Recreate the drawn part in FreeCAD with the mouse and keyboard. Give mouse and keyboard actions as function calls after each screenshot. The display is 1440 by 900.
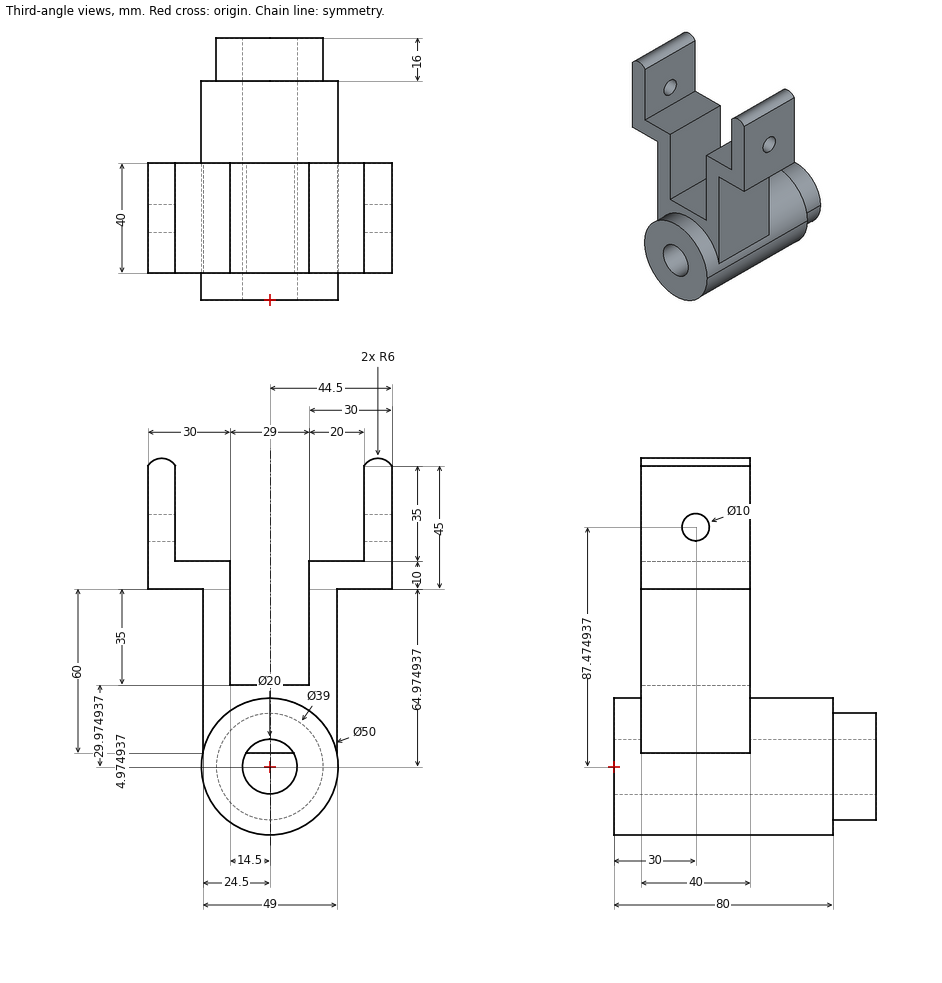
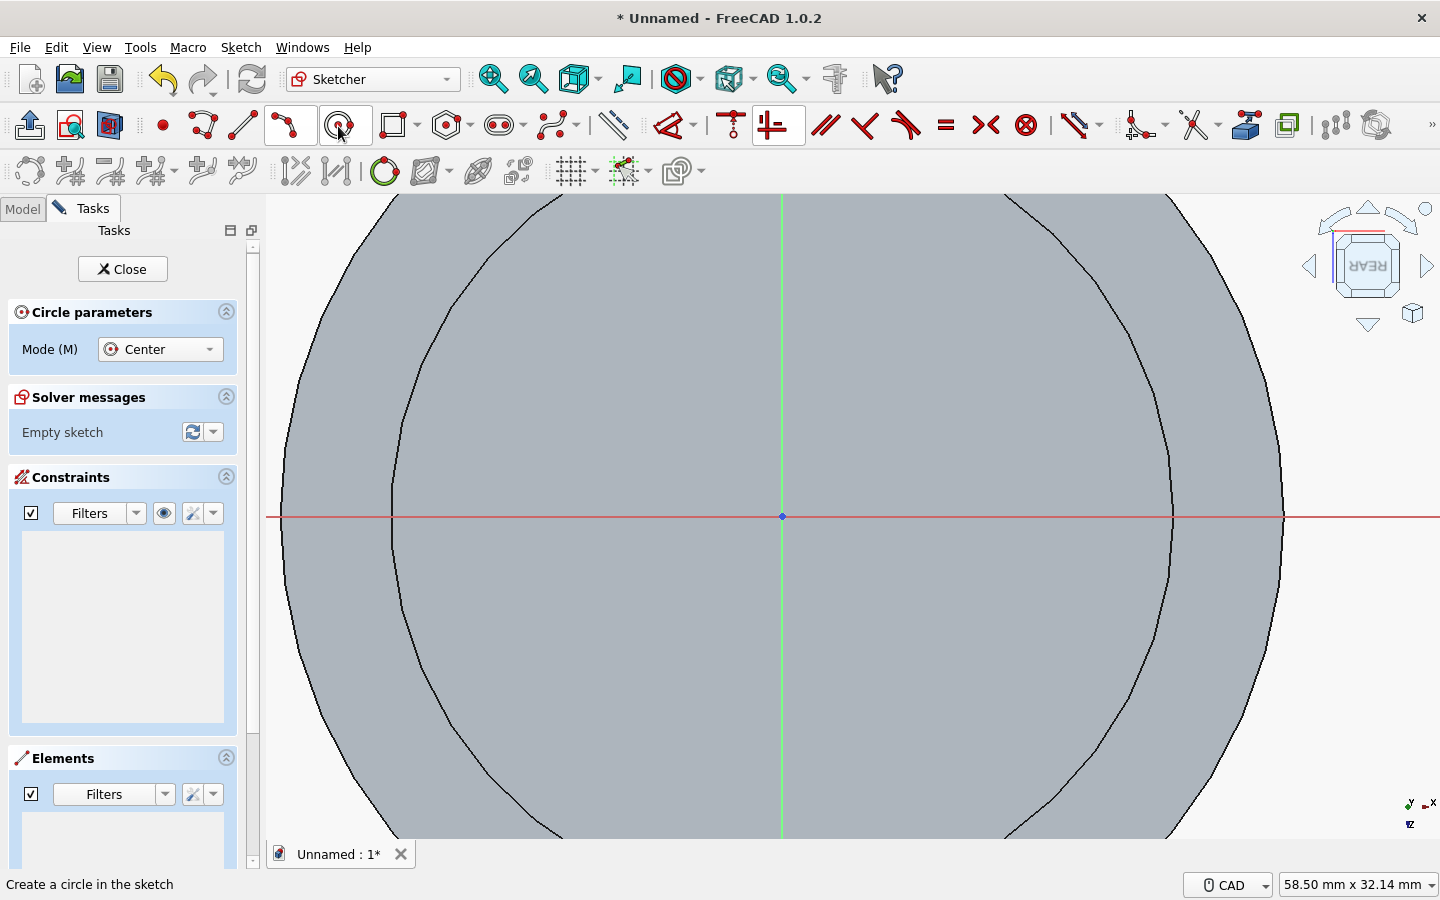
click(782, 516)
click(924, 375)
key(Escape)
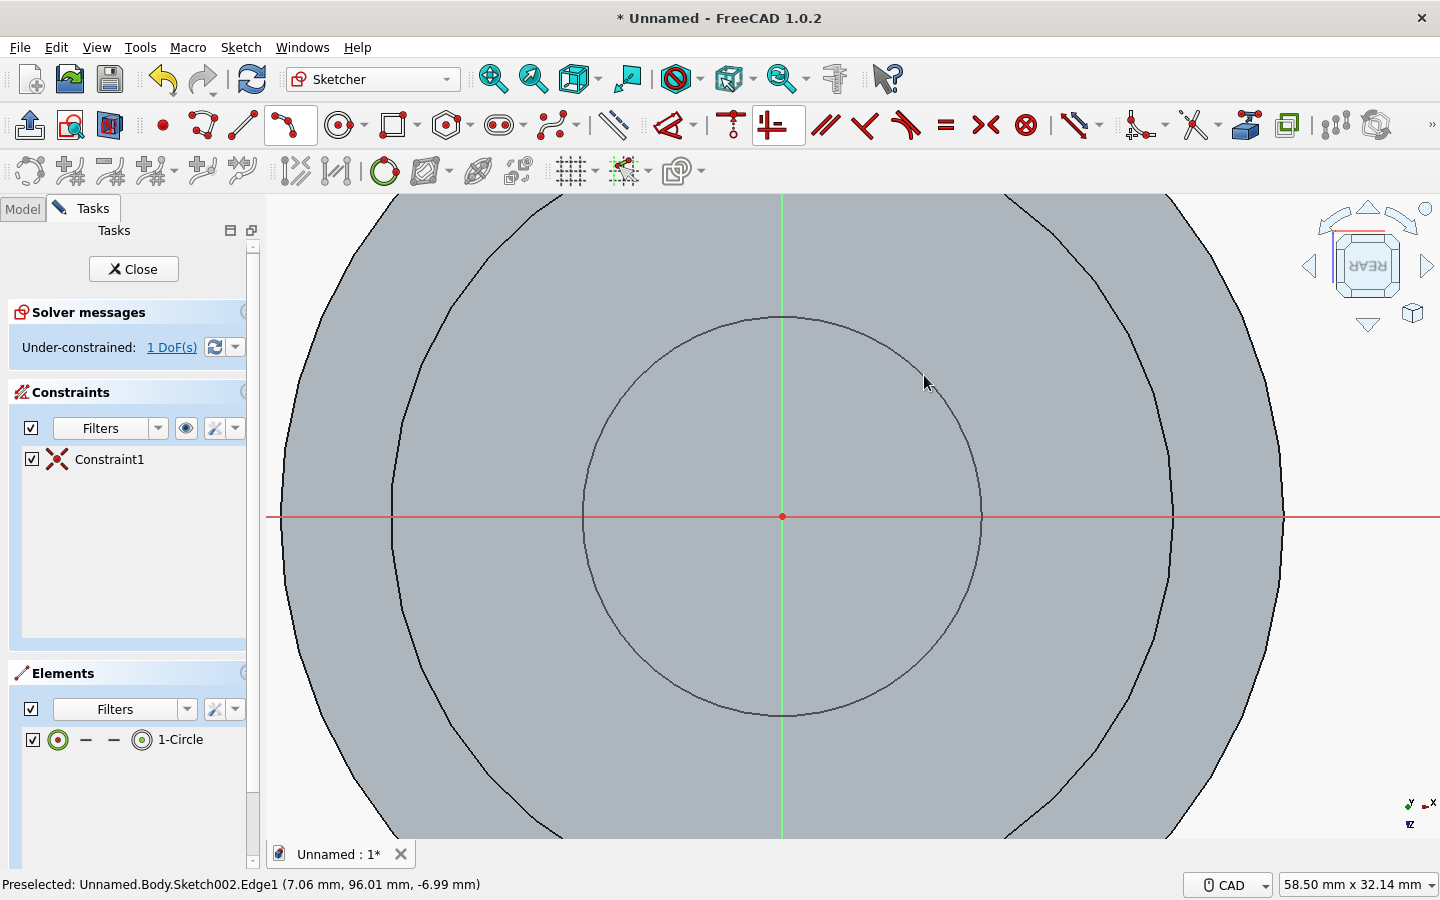
click(668, 126)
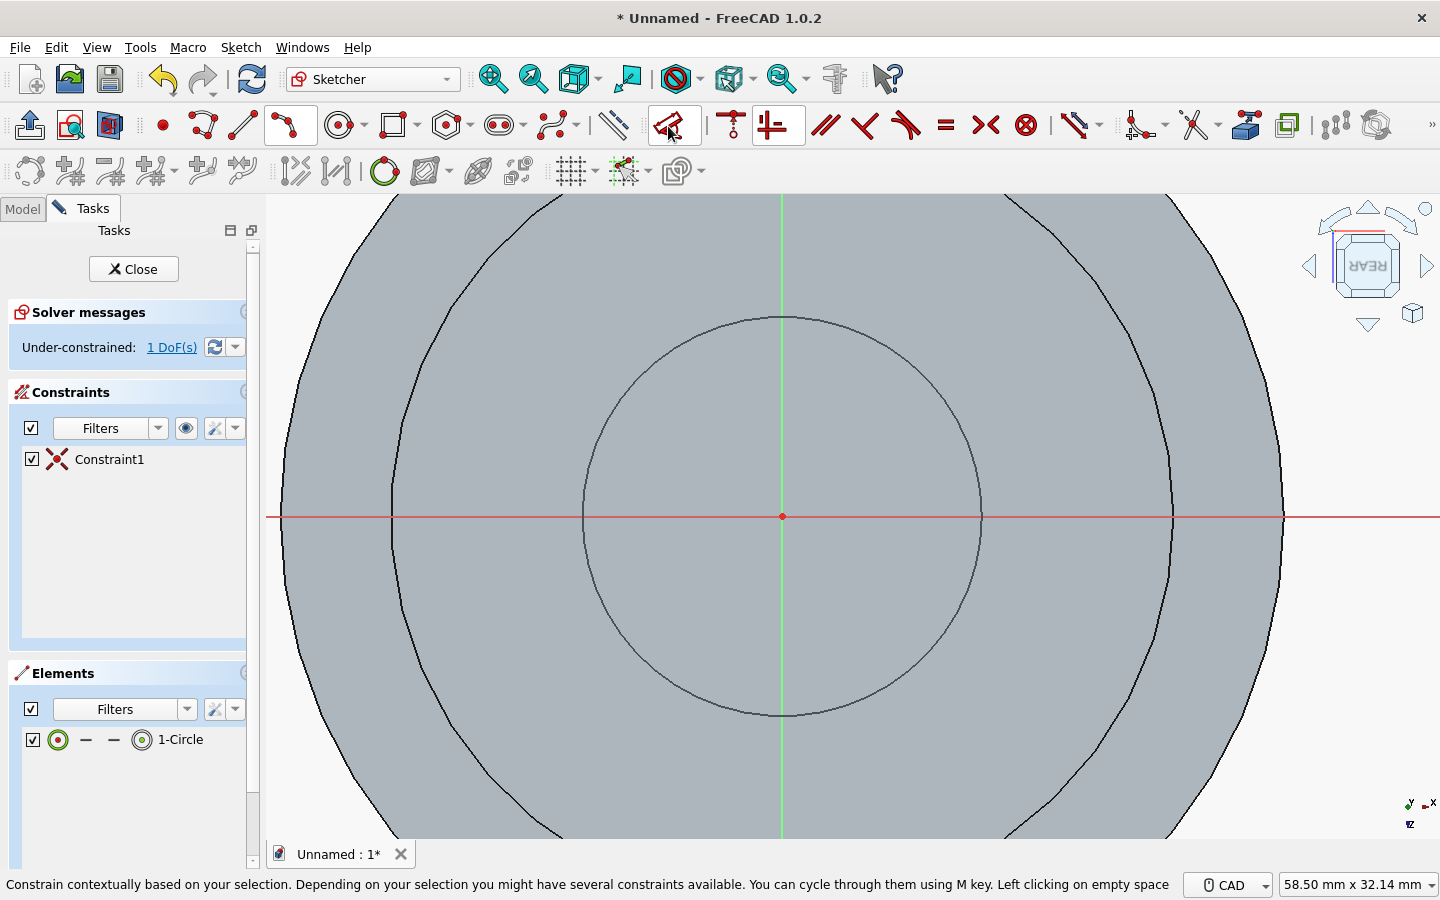
click(923, 375)
click(946, 352)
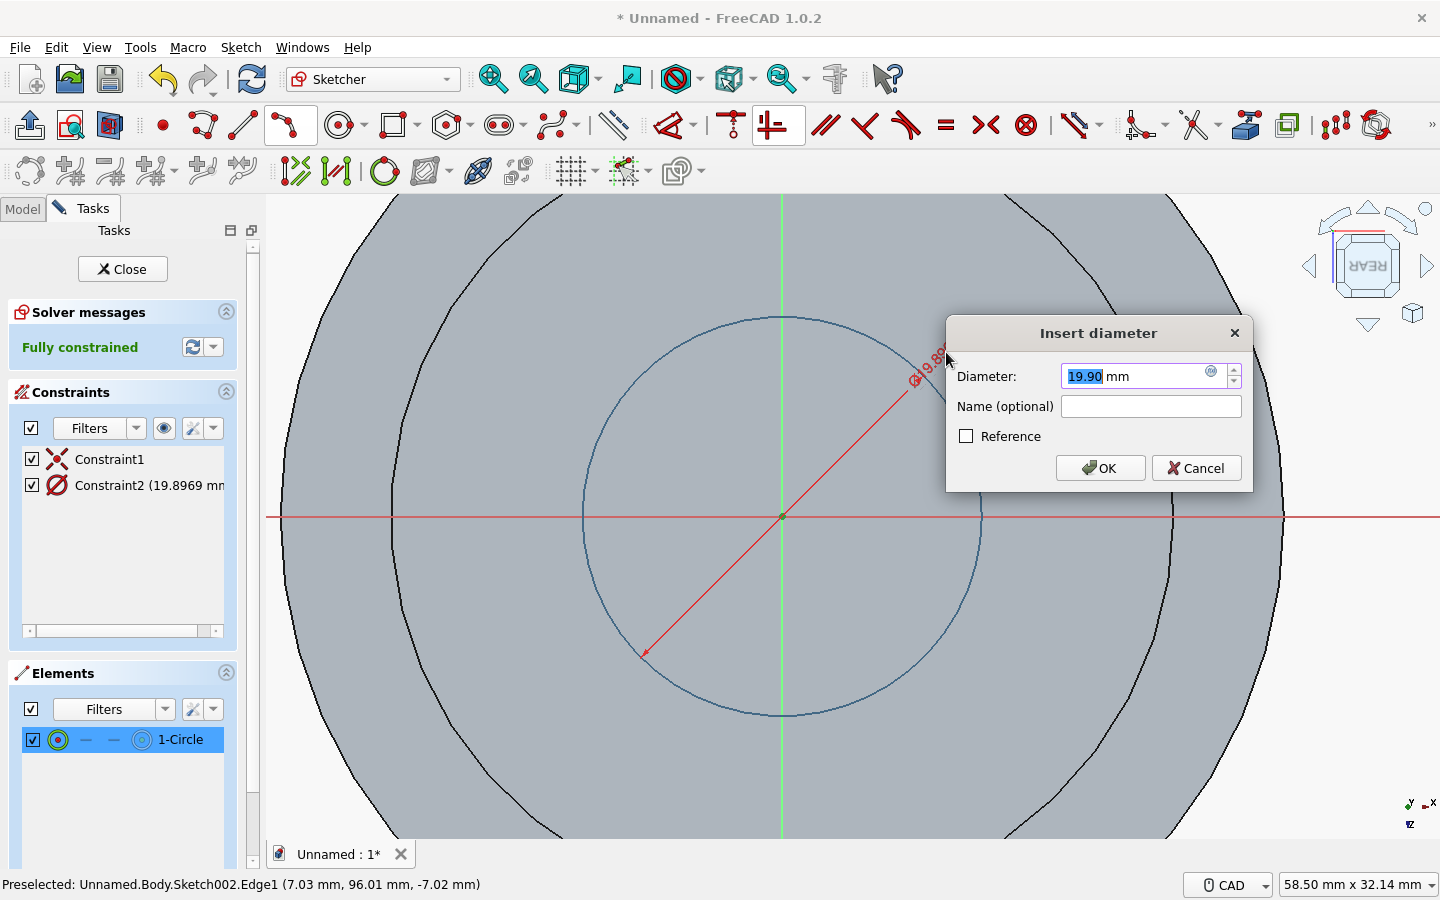
text(20)
key(Return)
key(Escape)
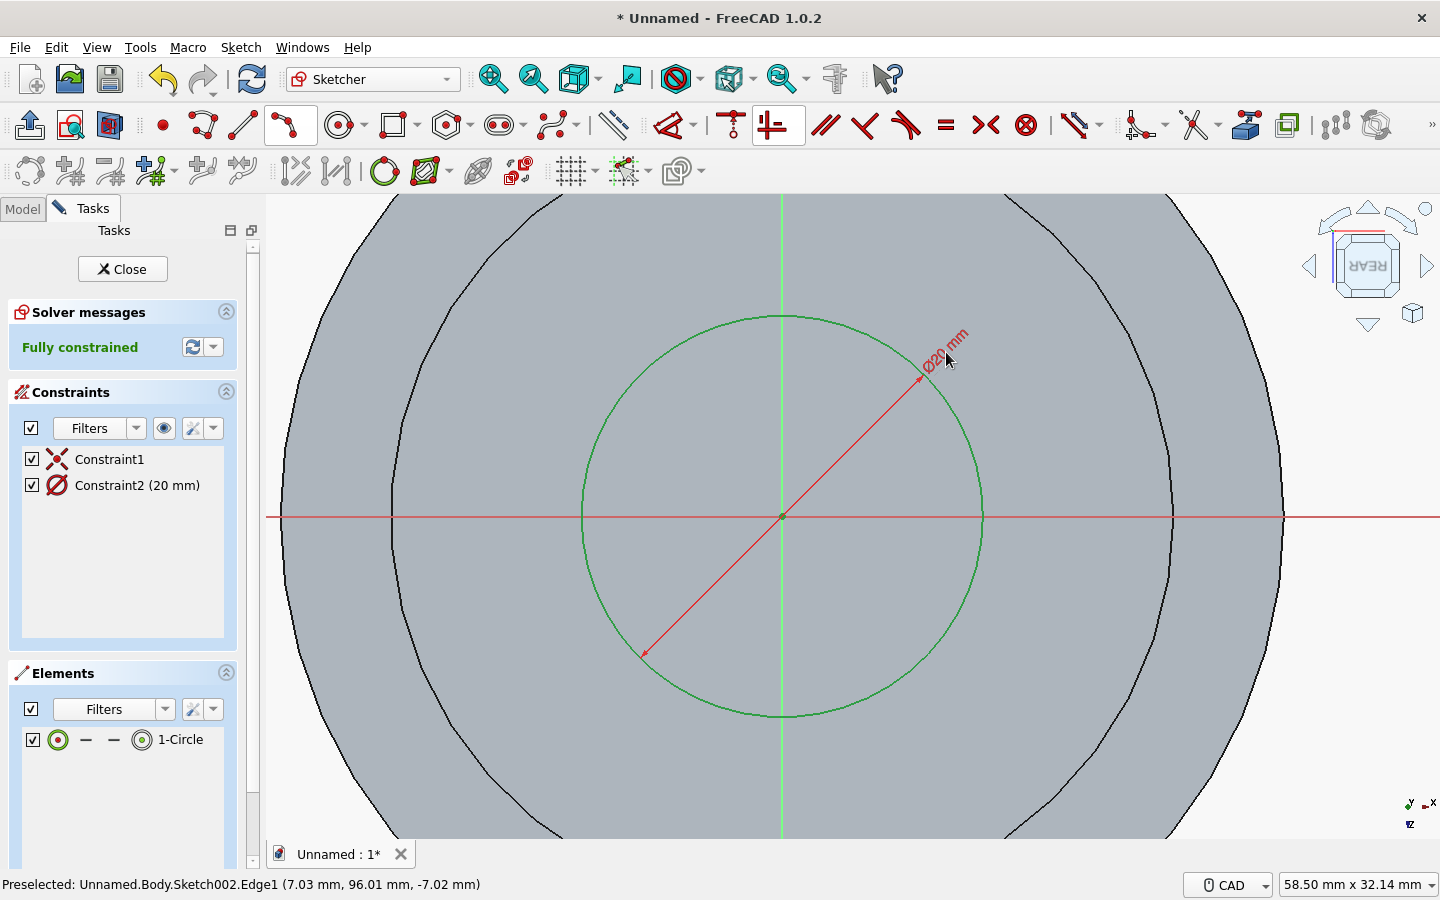
click(123, 269)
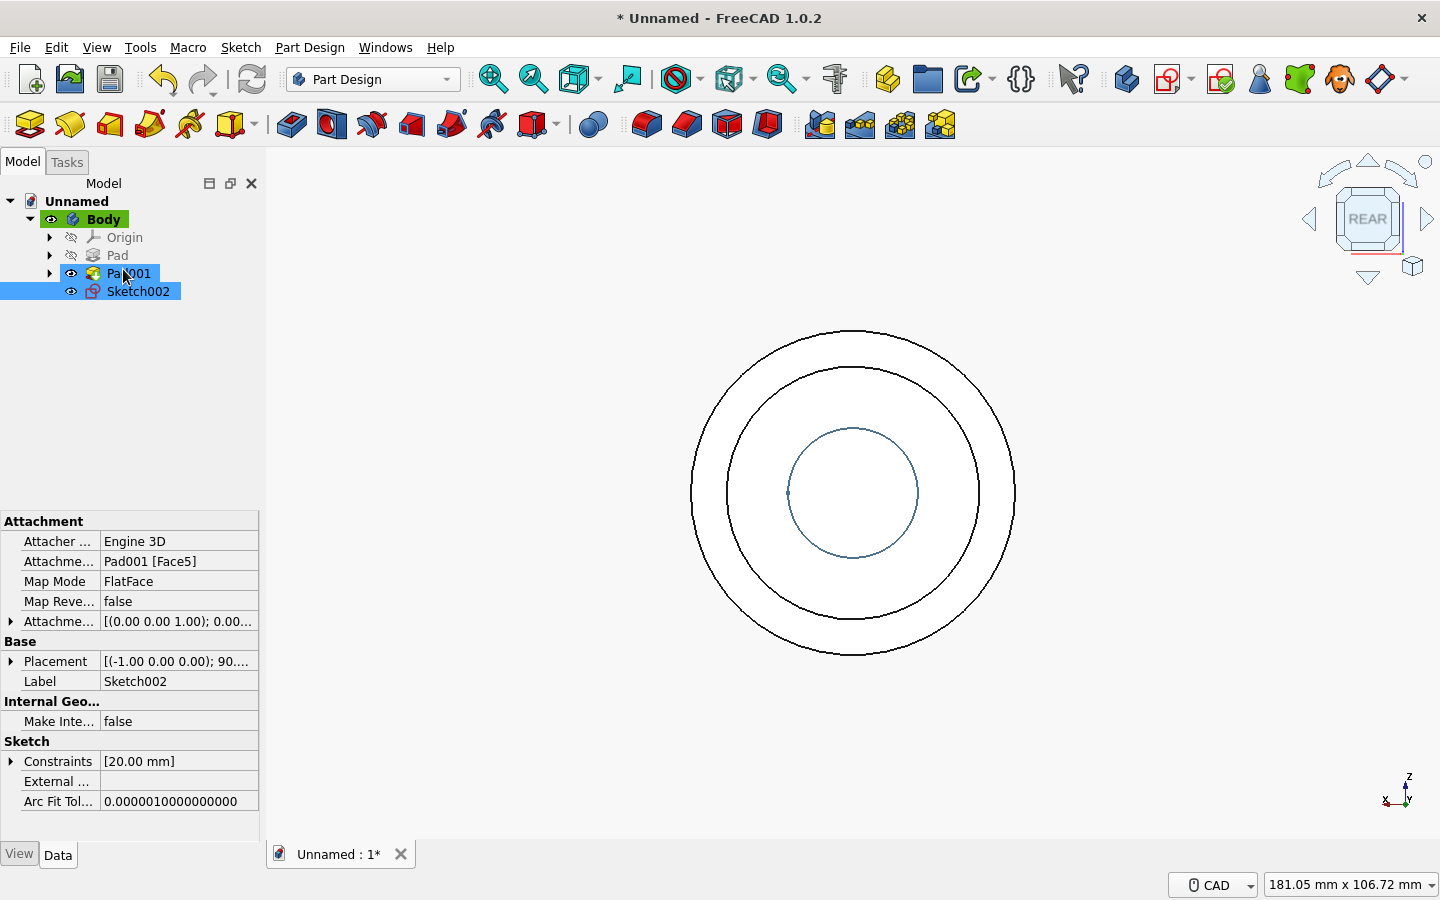
click(292, 124)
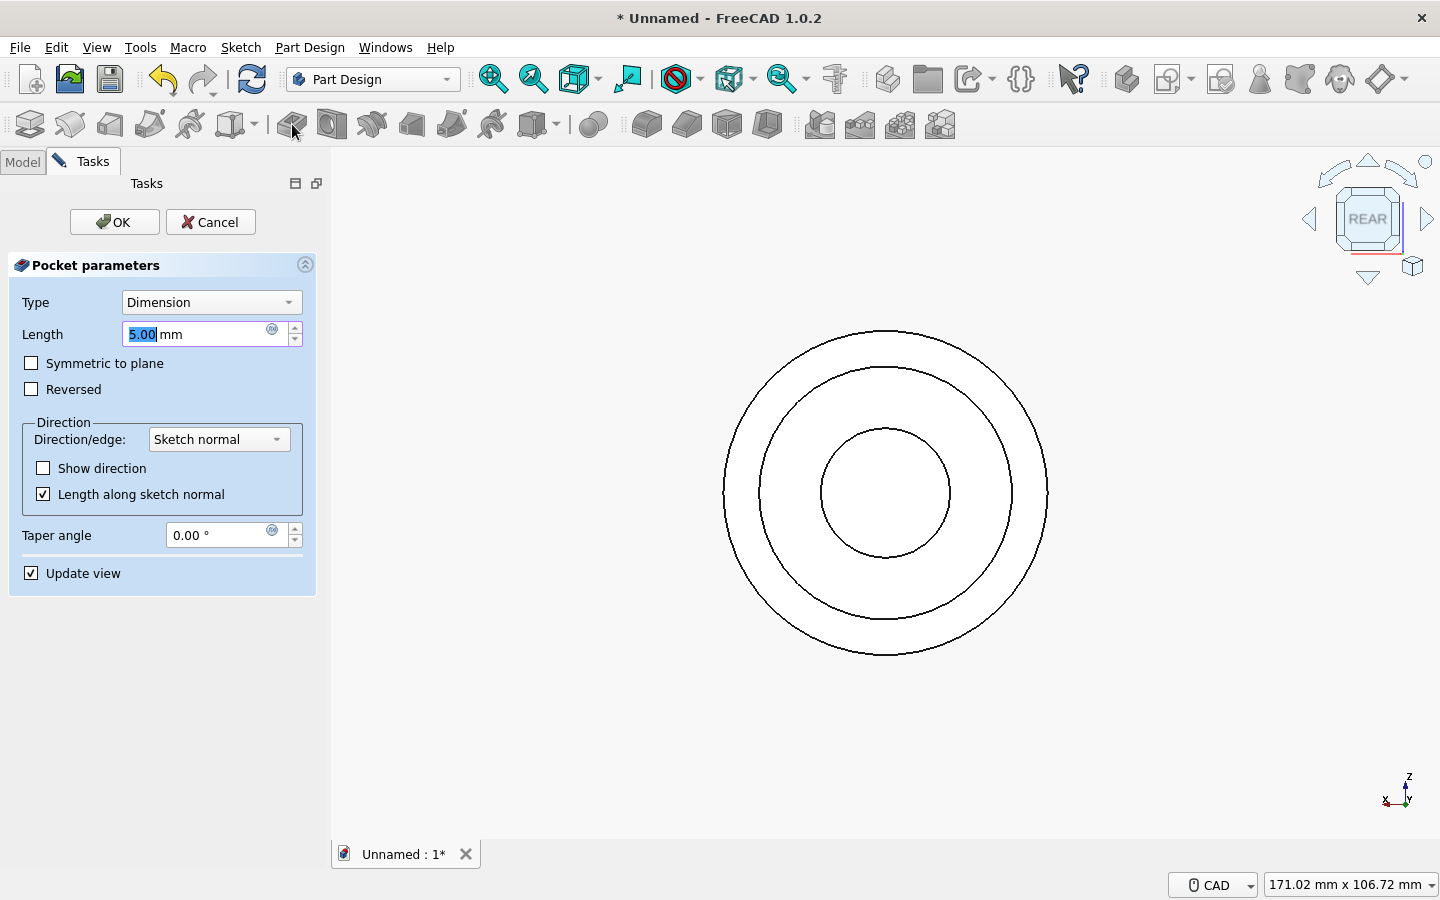
click(212, 302)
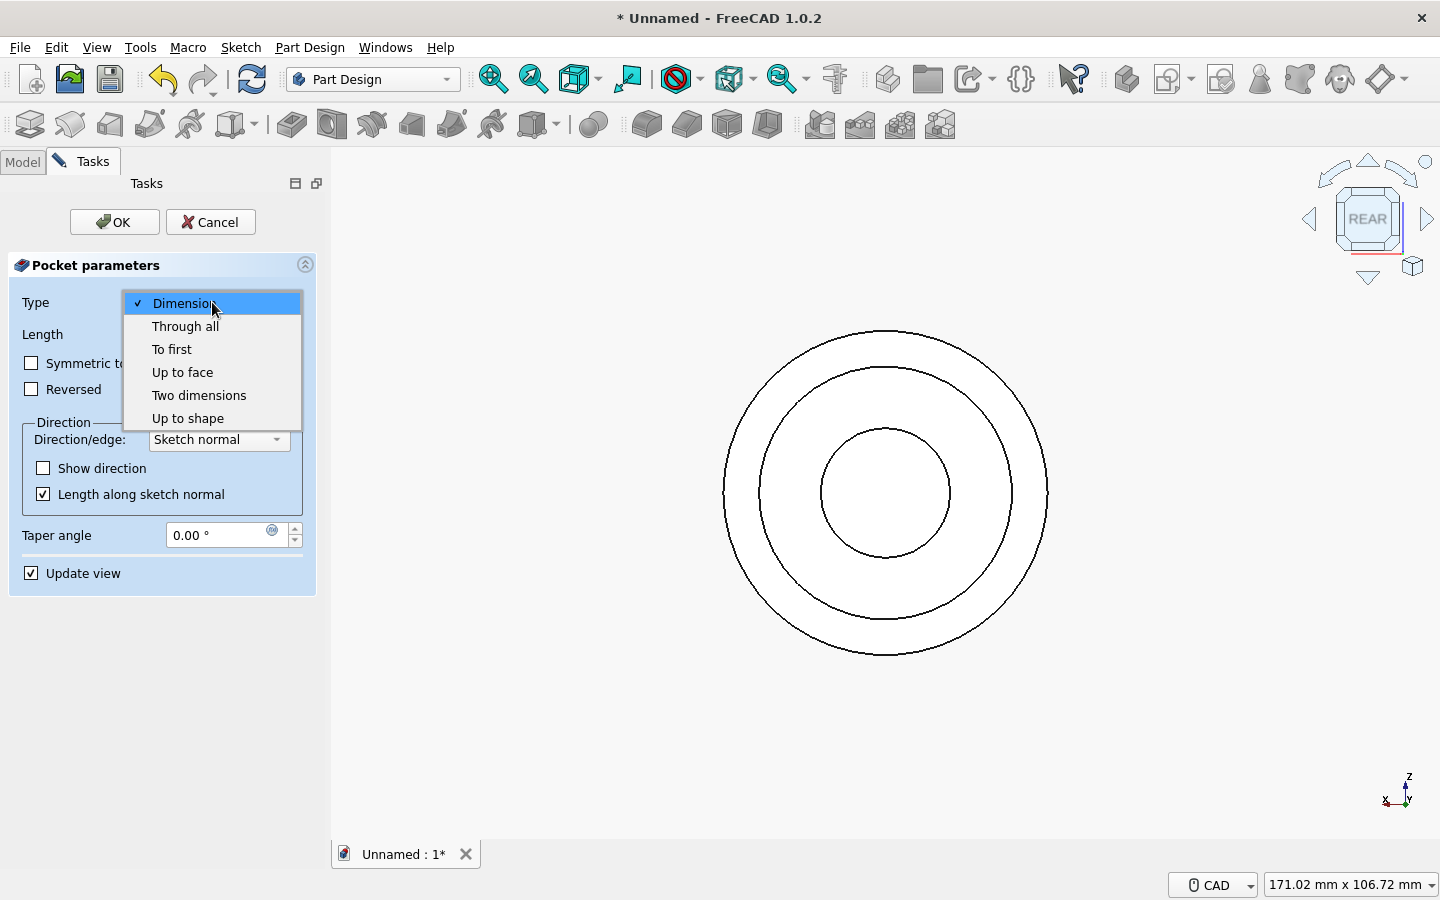
click(212, 326)